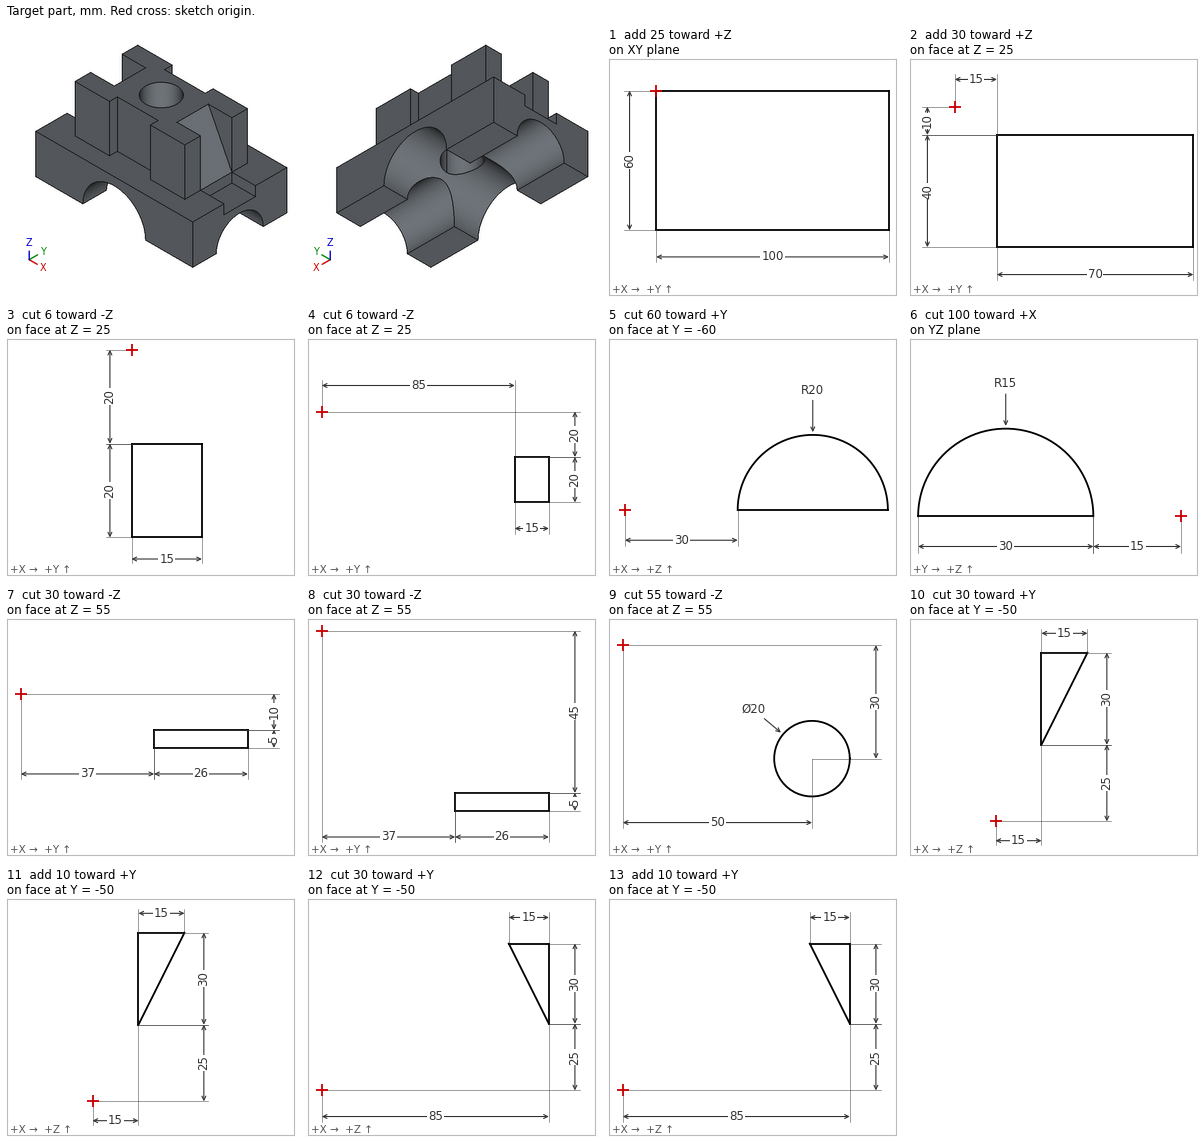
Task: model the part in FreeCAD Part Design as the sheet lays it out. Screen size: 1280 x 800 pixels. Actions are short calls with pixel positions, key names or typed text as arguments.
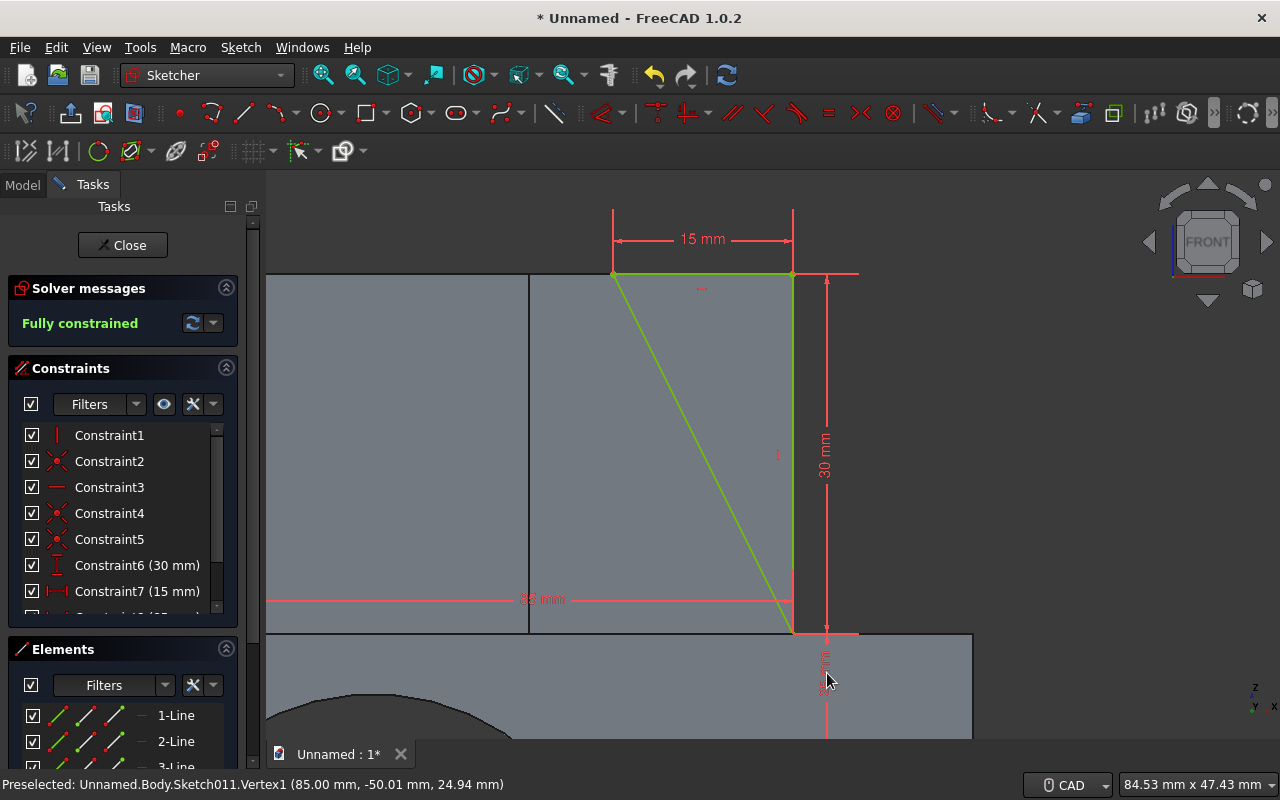
click(123, 245)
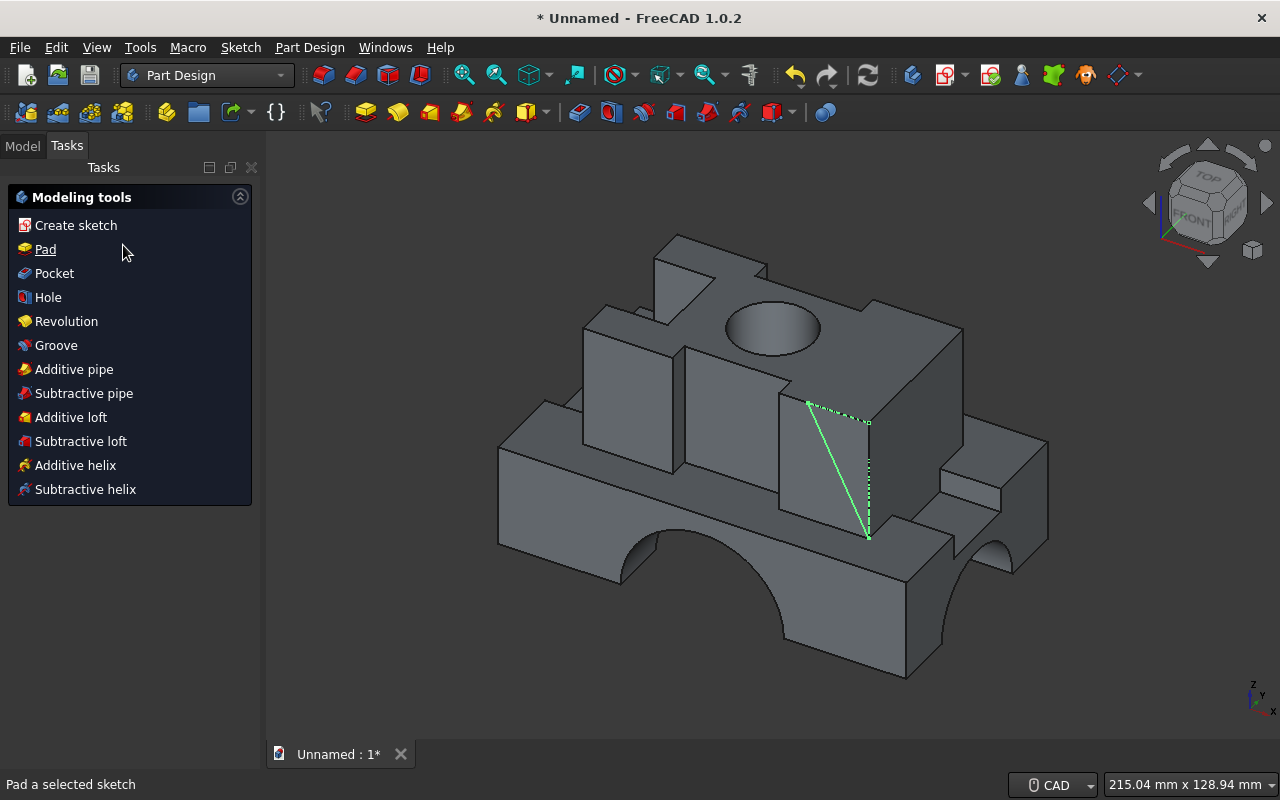
click(580, 112)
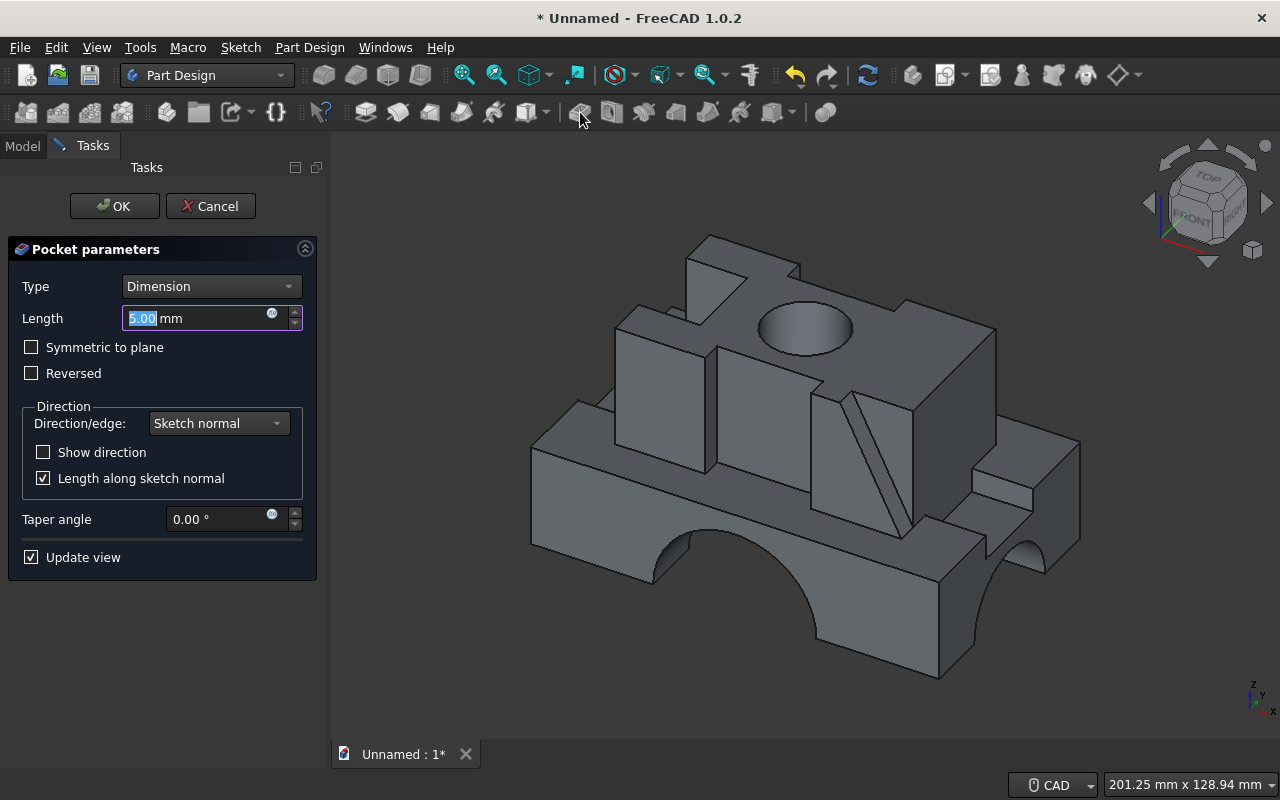
text(30)
key(Tab)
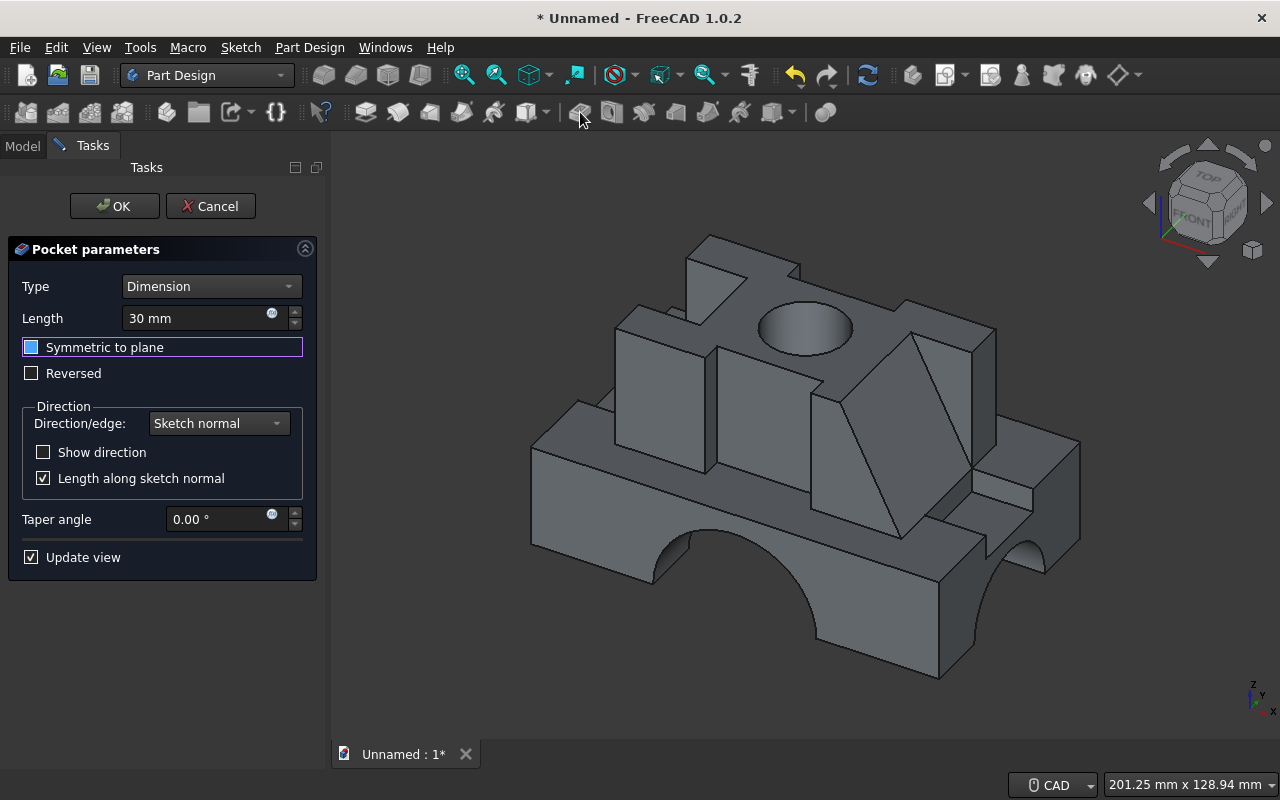
click(115, 206)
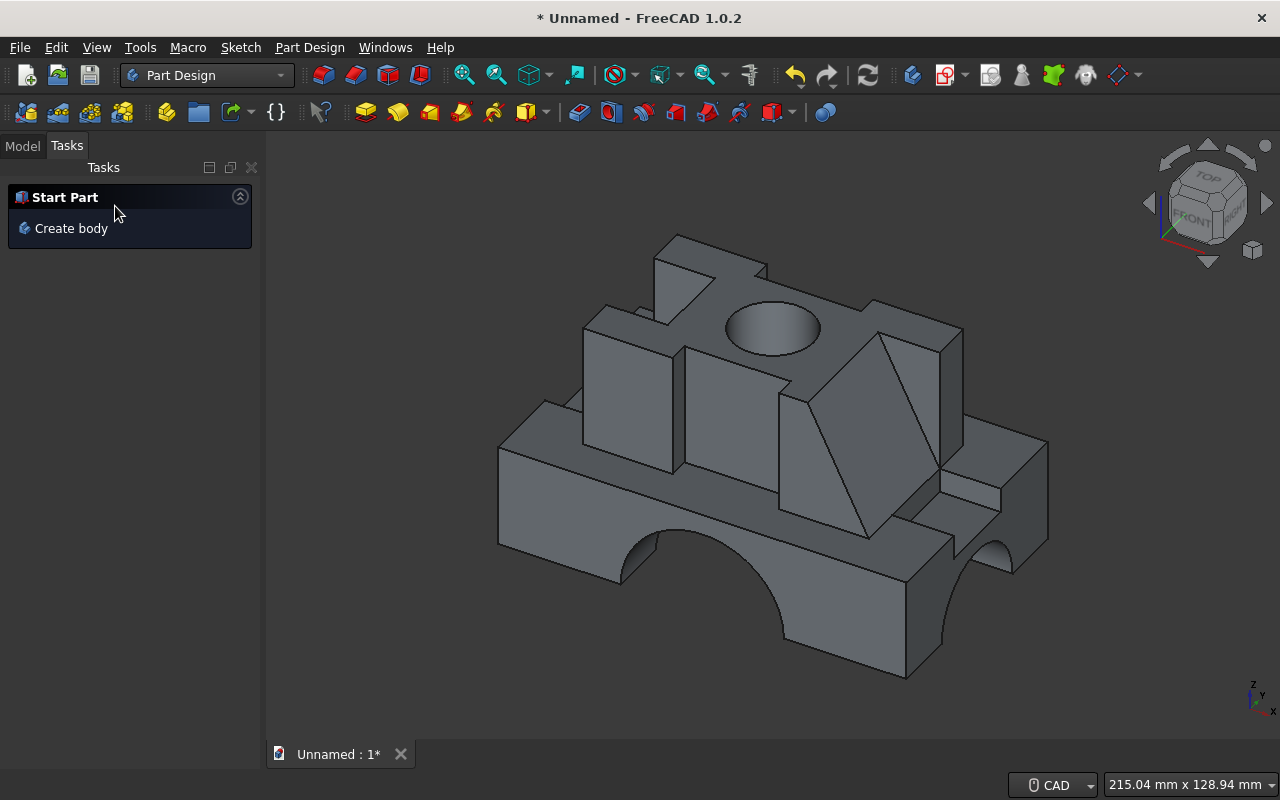
click(628, 400)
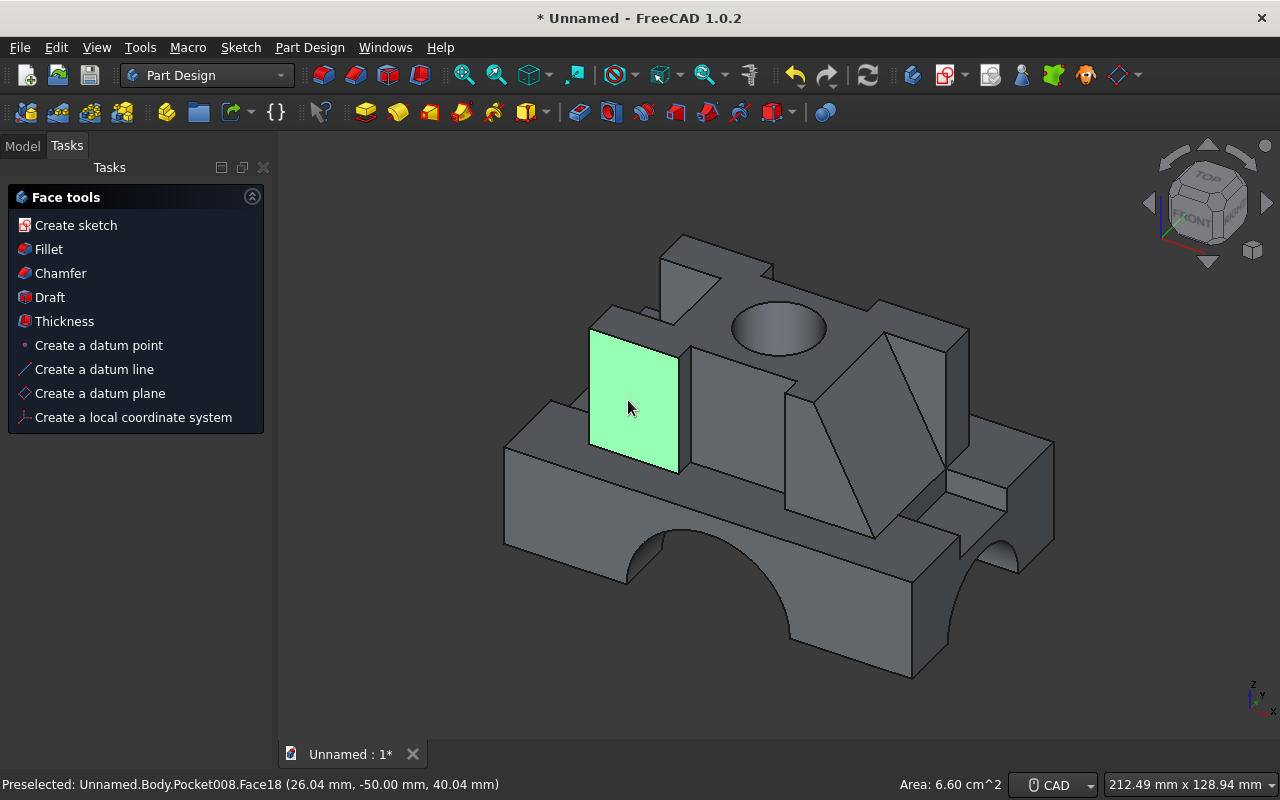
click(946, 76)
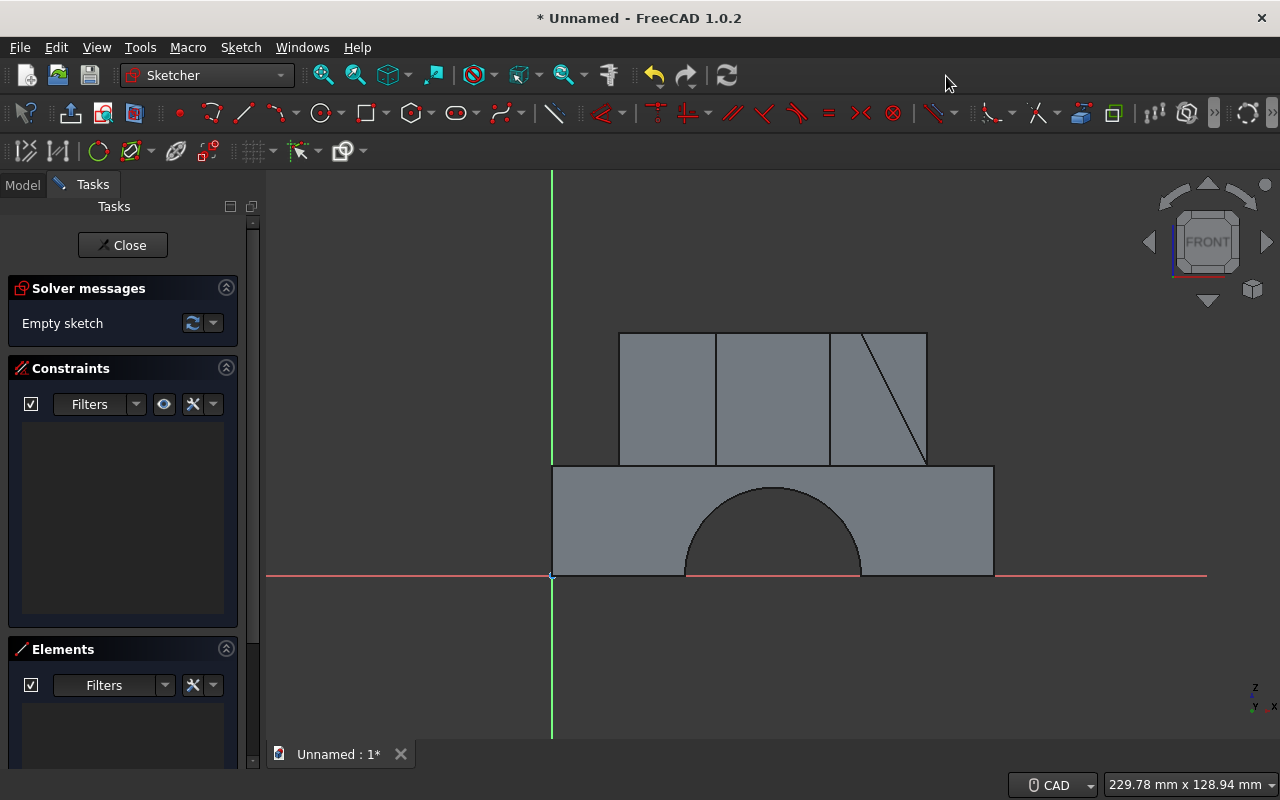
scroll(1005, 367, up, 5)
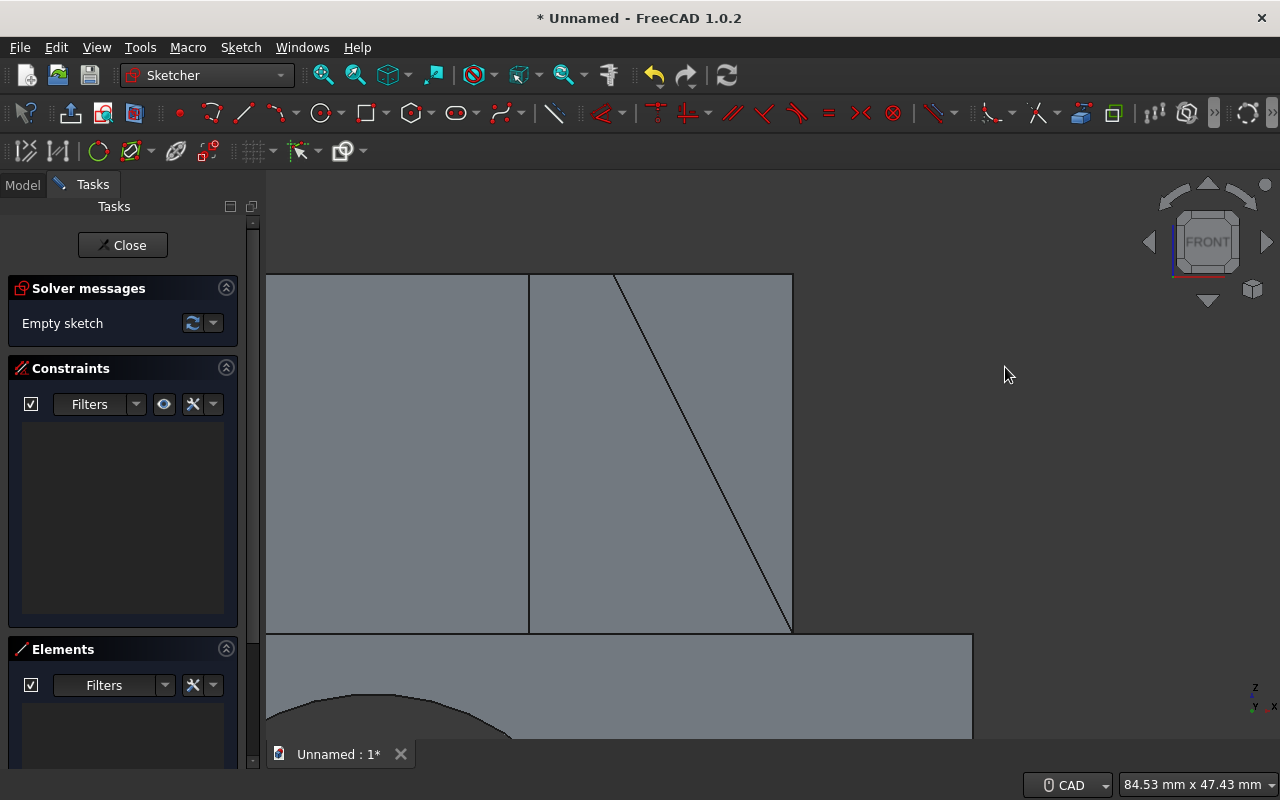
click(212, 114)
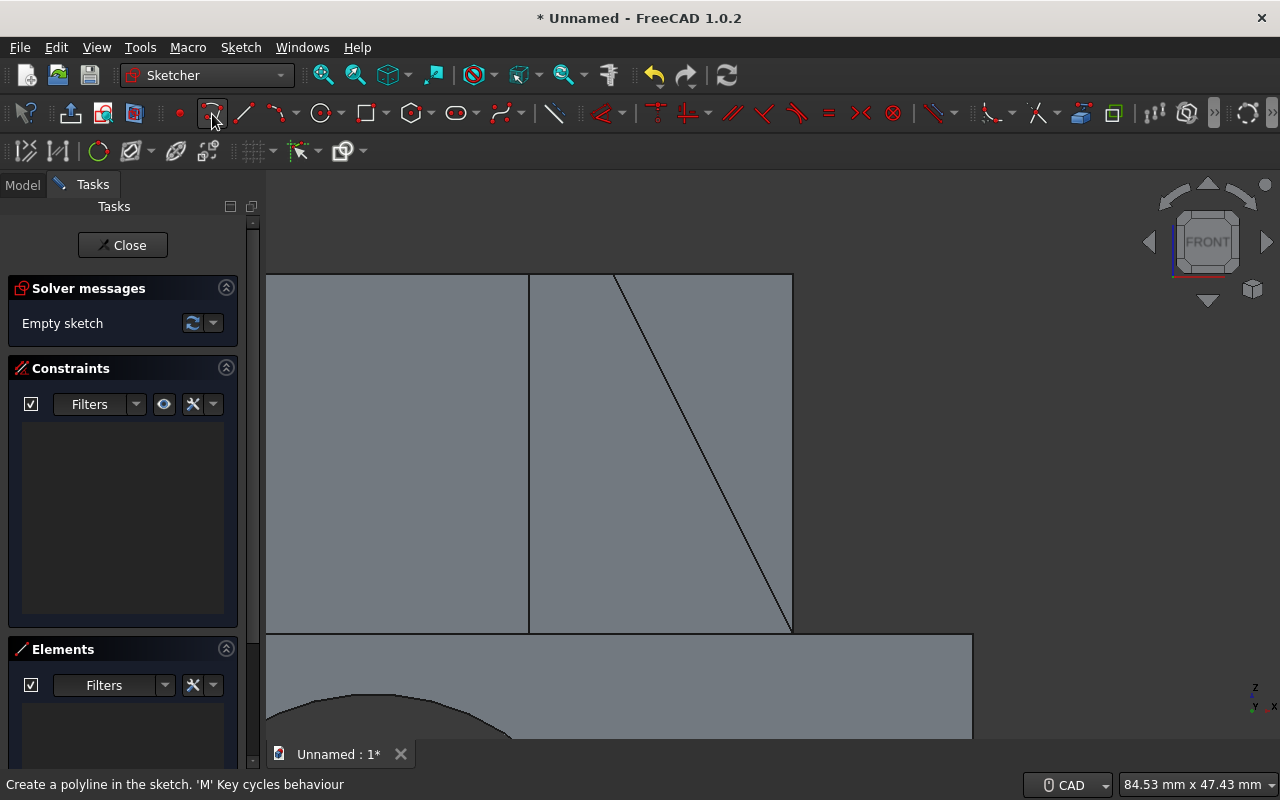
click(793, 634)
click(793, 274)
click(613, 274)
click(793, 635)
key(Escape)
key(Escape)